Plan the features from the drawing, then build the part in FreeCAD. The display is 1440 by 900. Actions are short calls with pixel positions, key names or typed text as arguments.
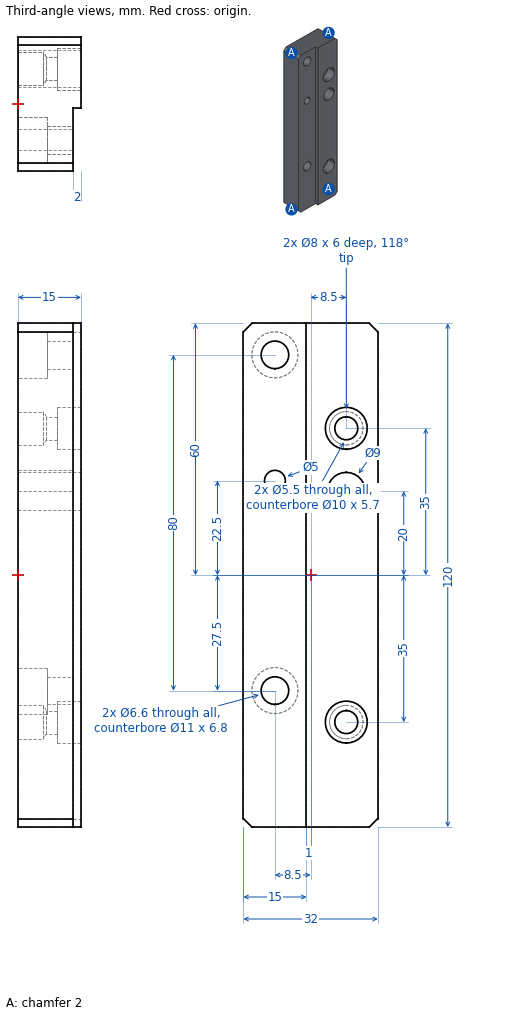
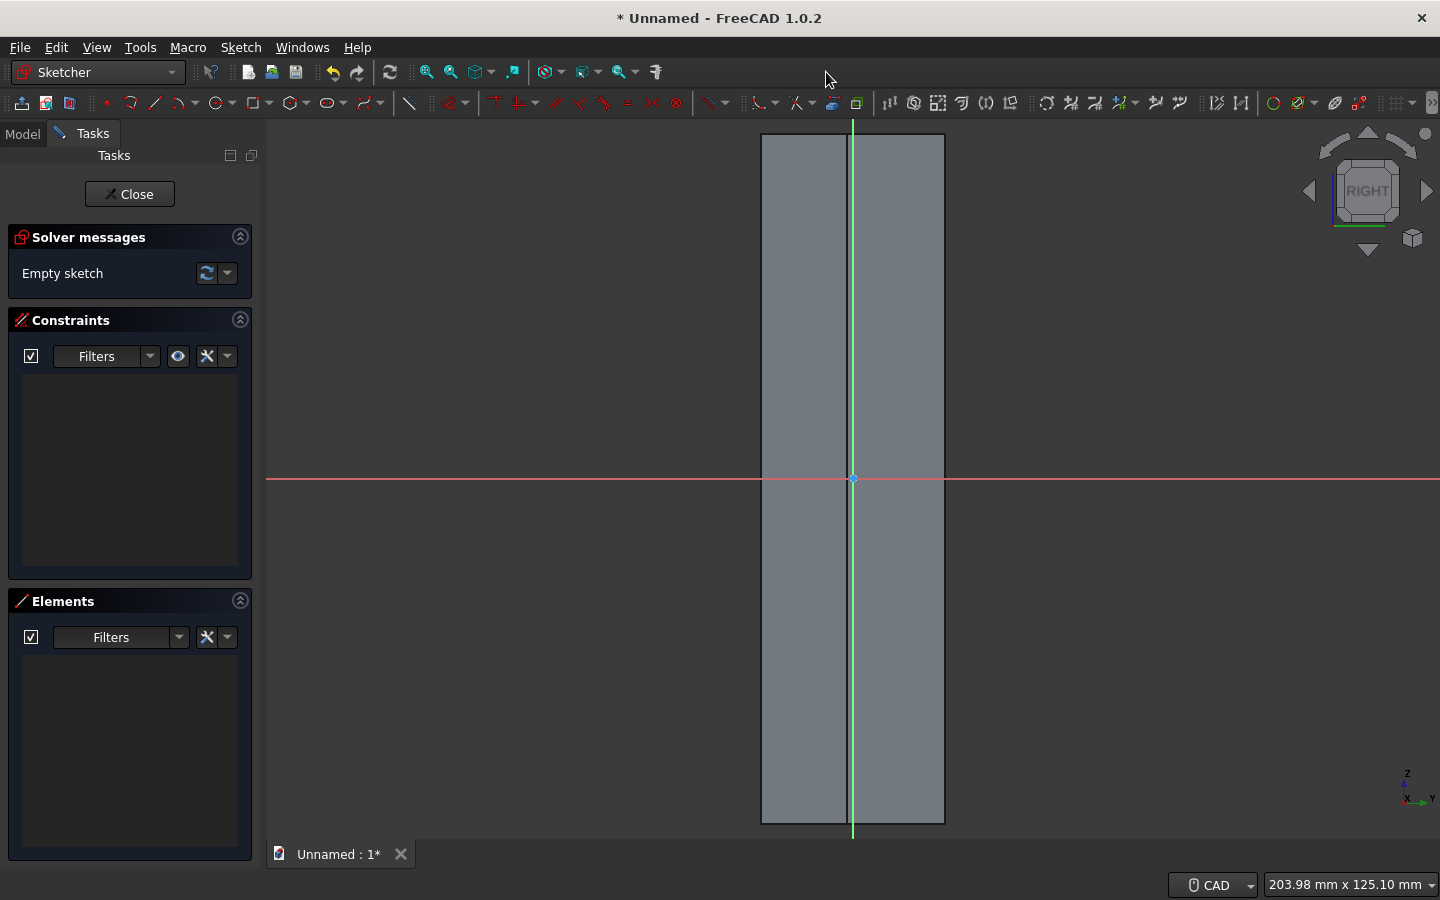
scroll(917, 350, up, 11)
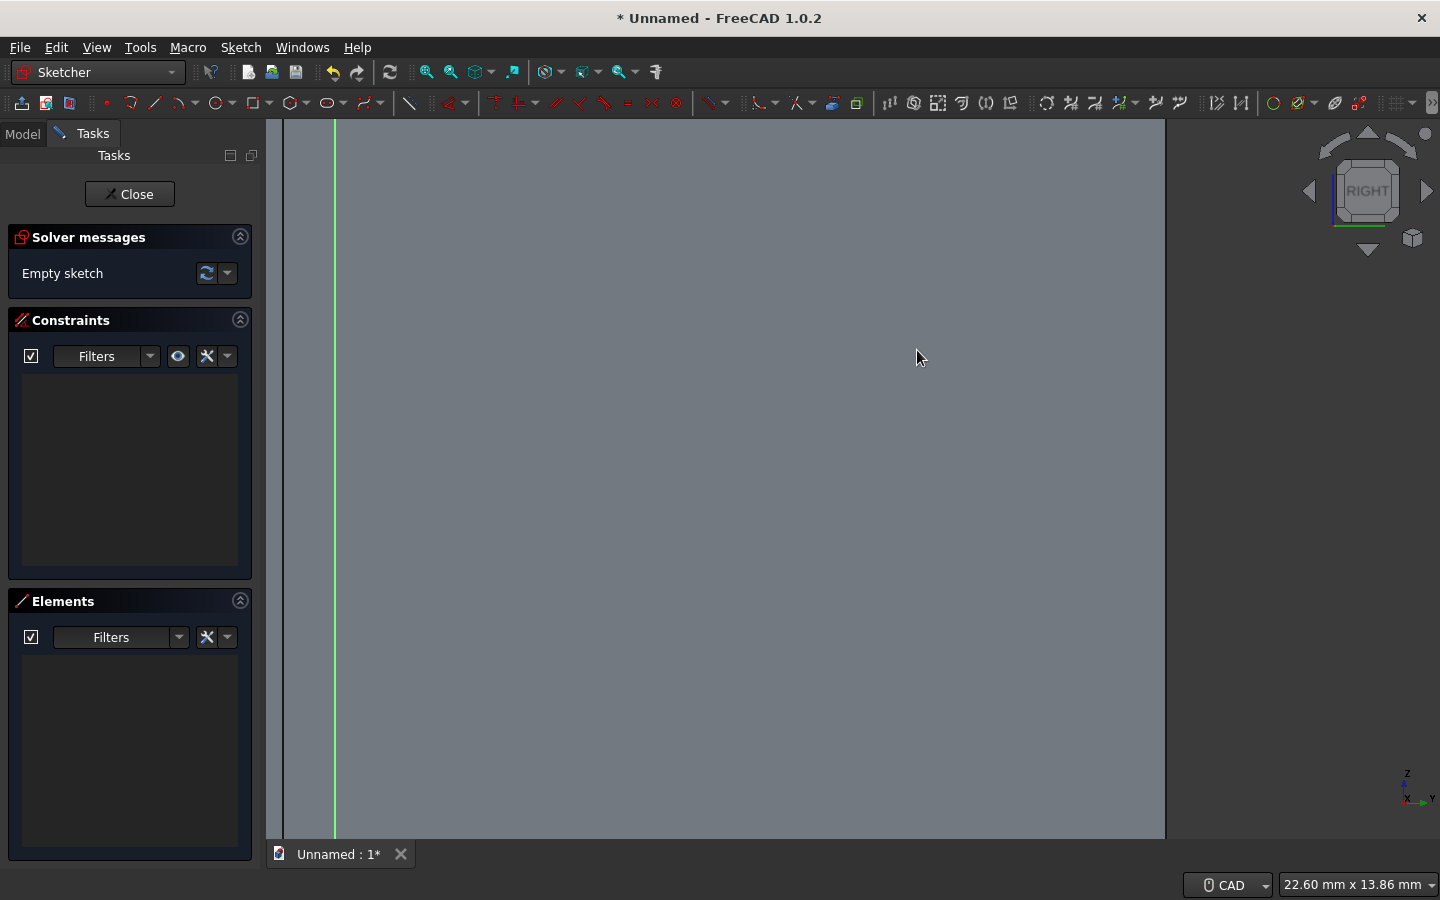
click(216, 104)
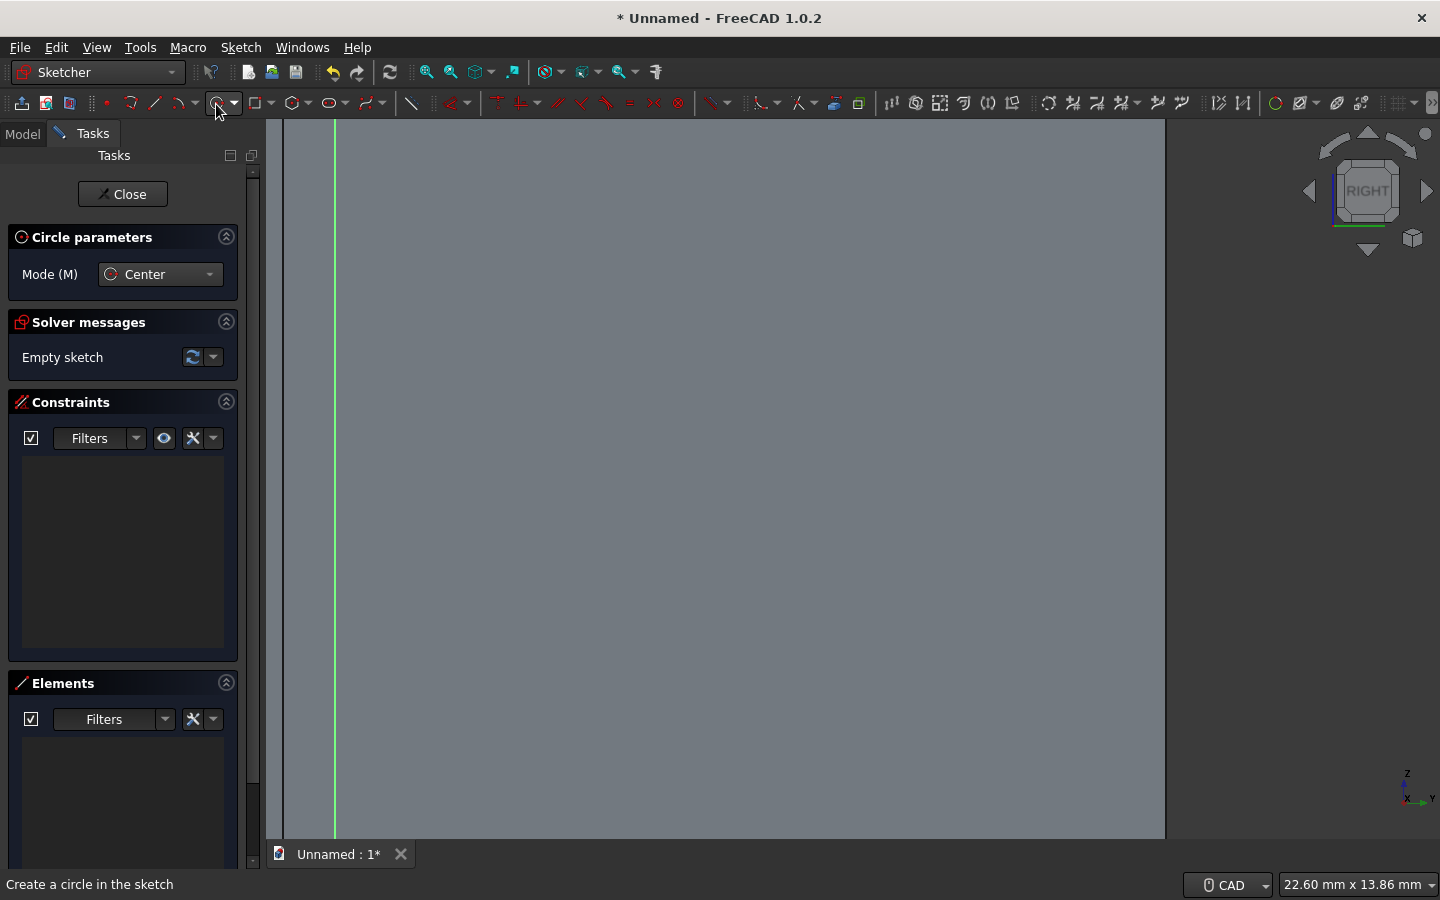
click(776, 473)
click(942, 307)
key(Escape)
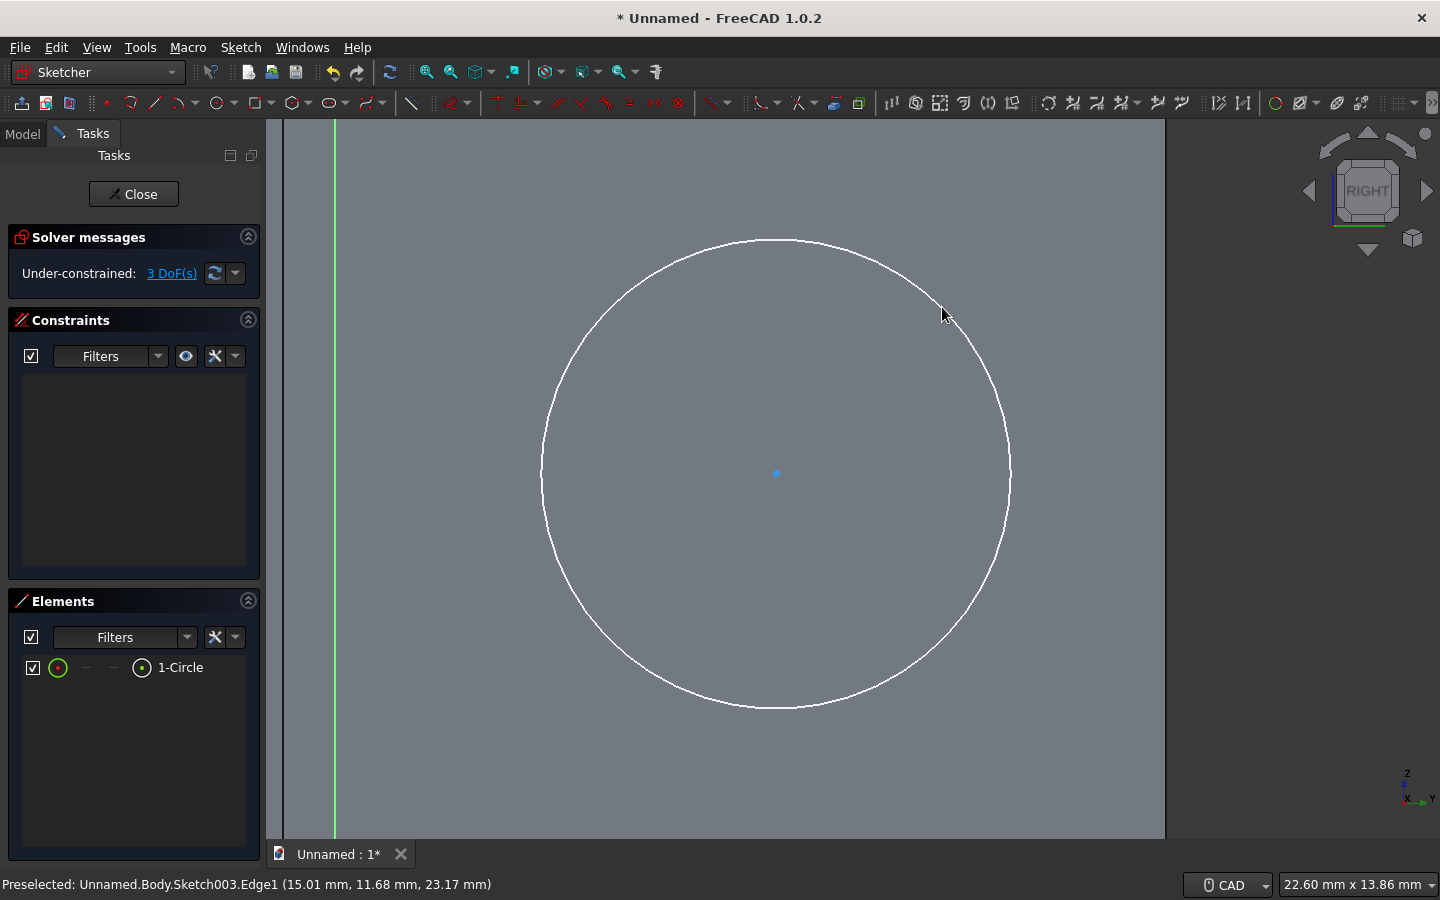
click(450, 104)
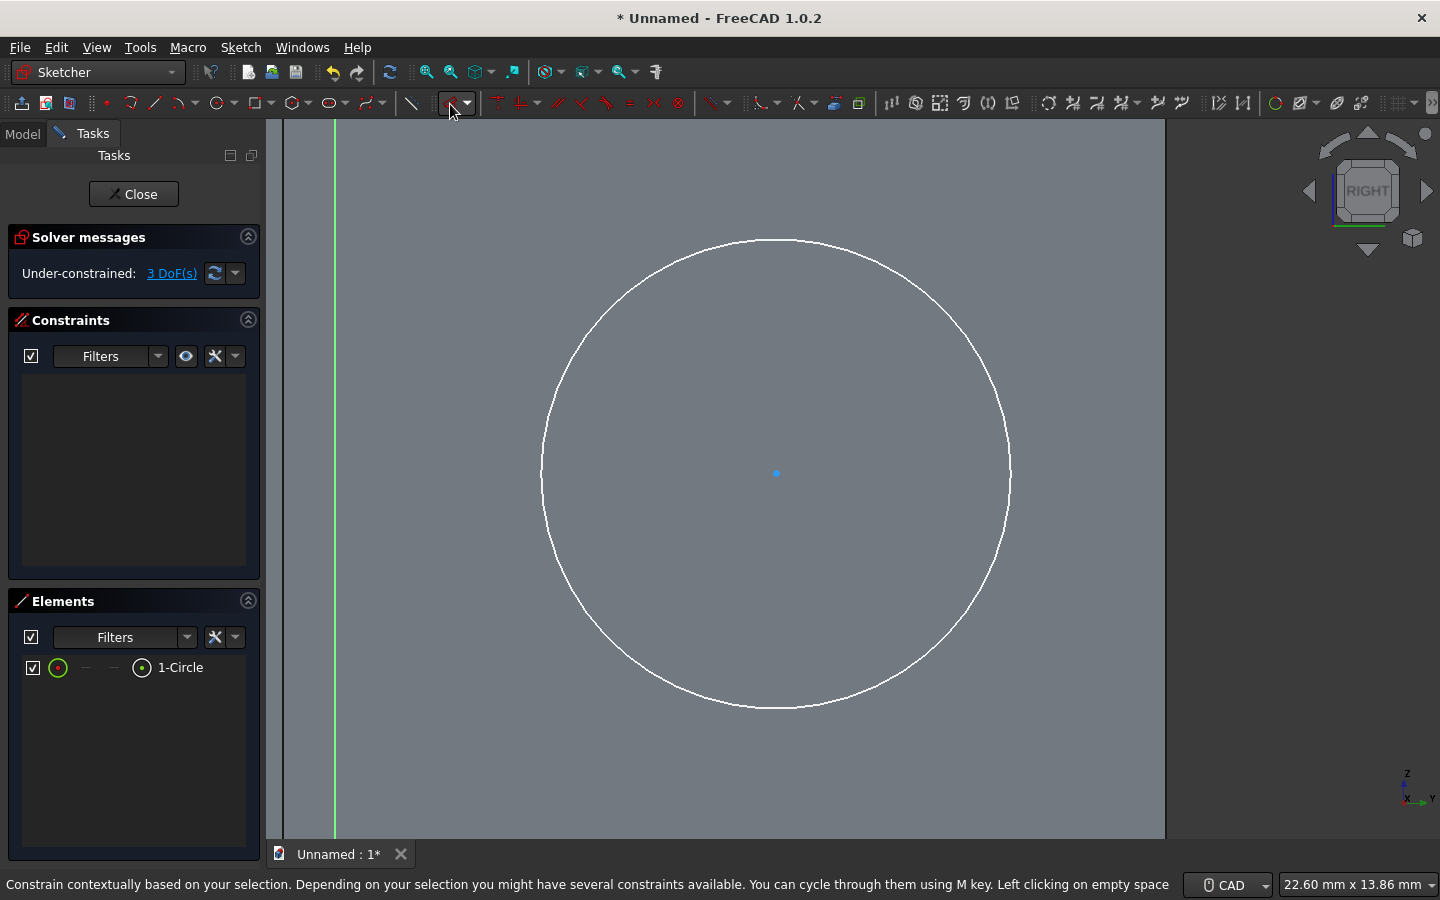
click(941, 307)
click(963, 284)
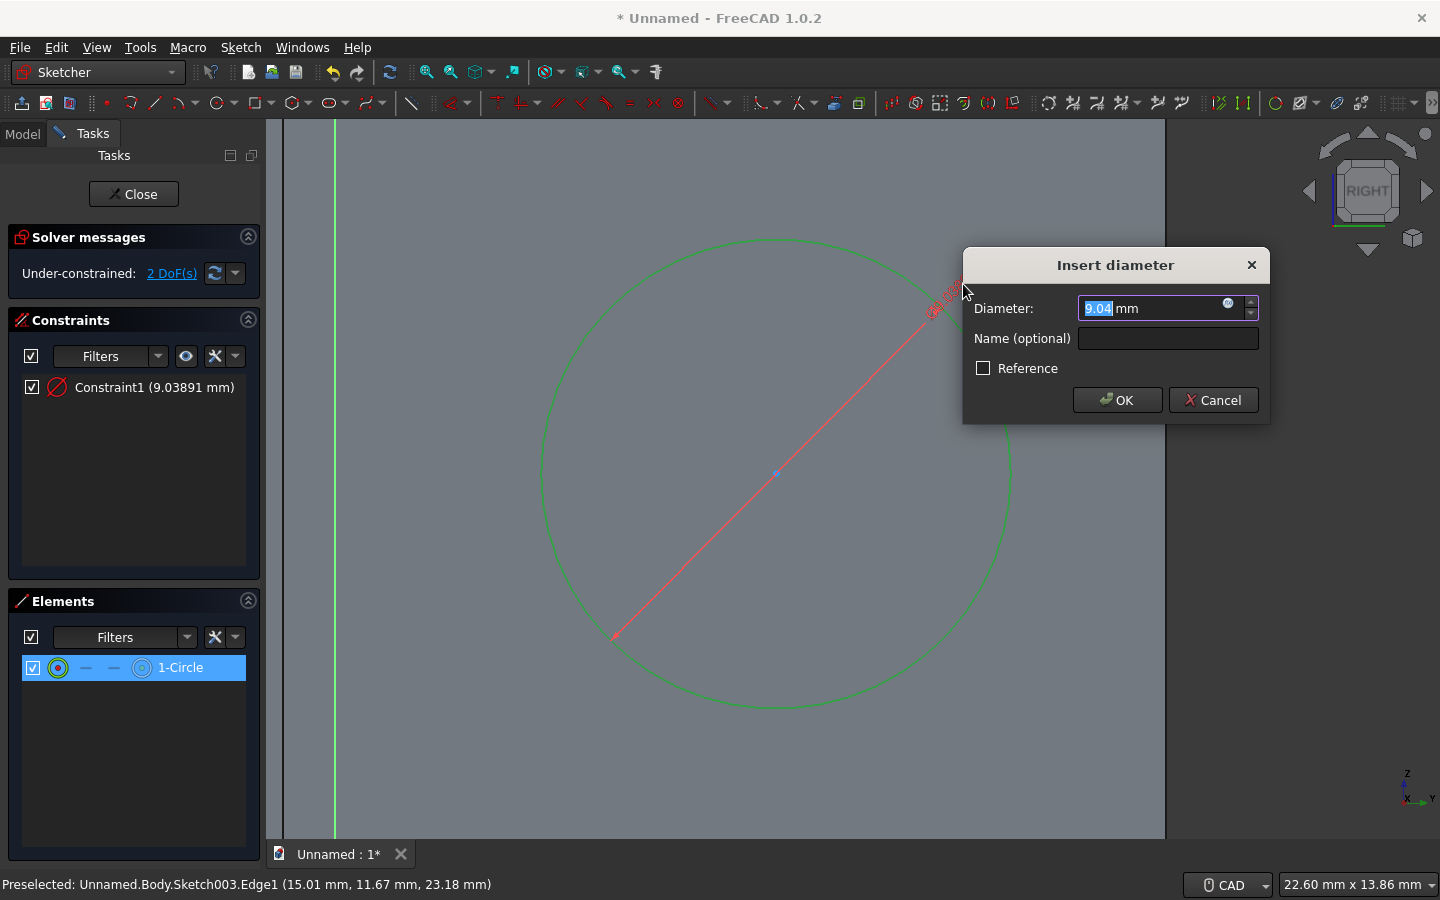
text(9)
key(Return)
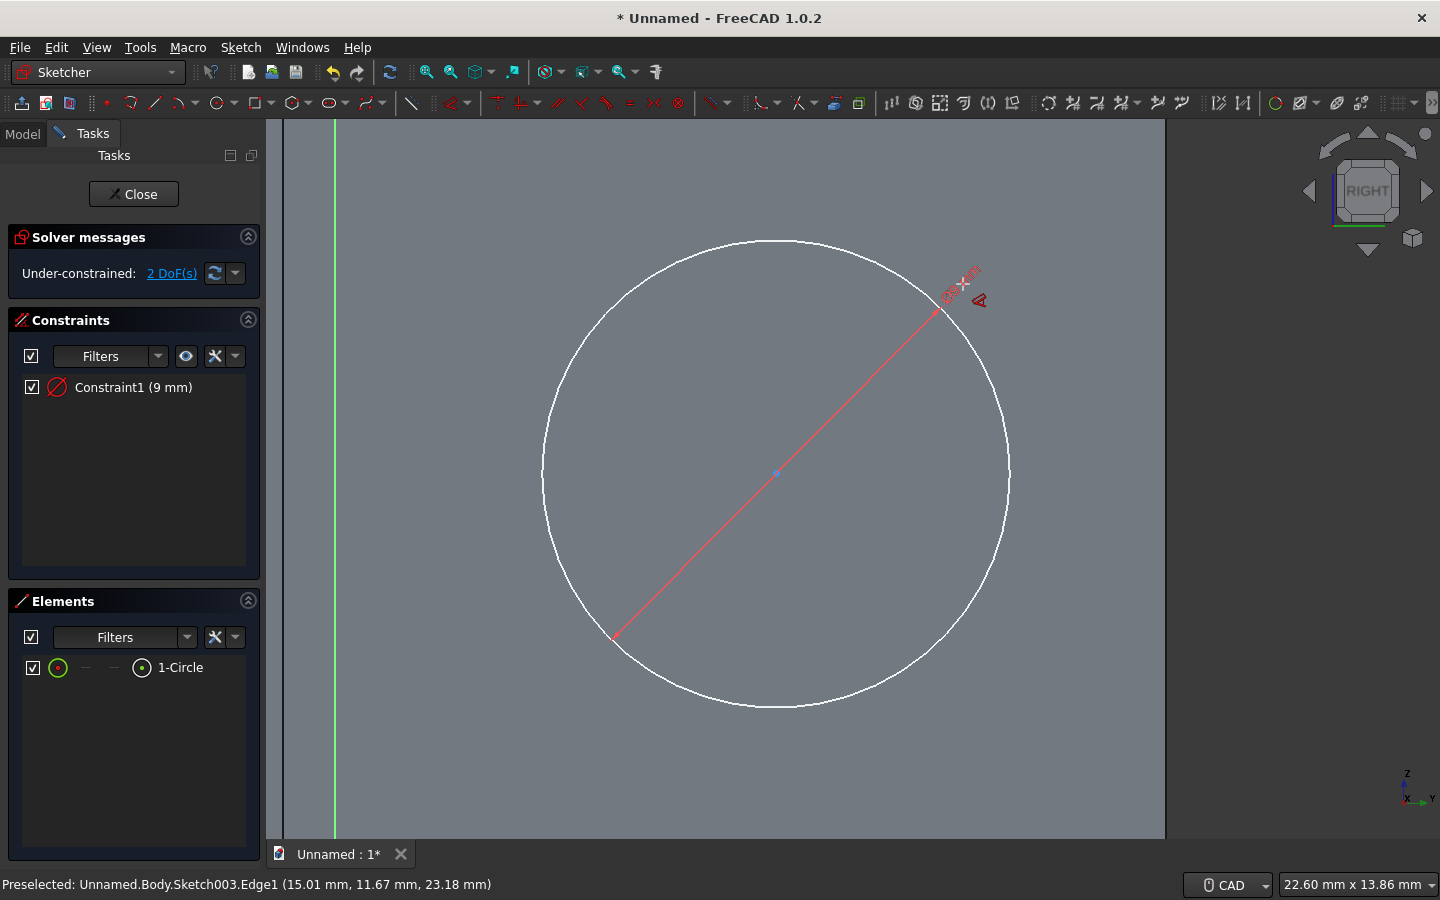
click(776, 474)
click(301, 643)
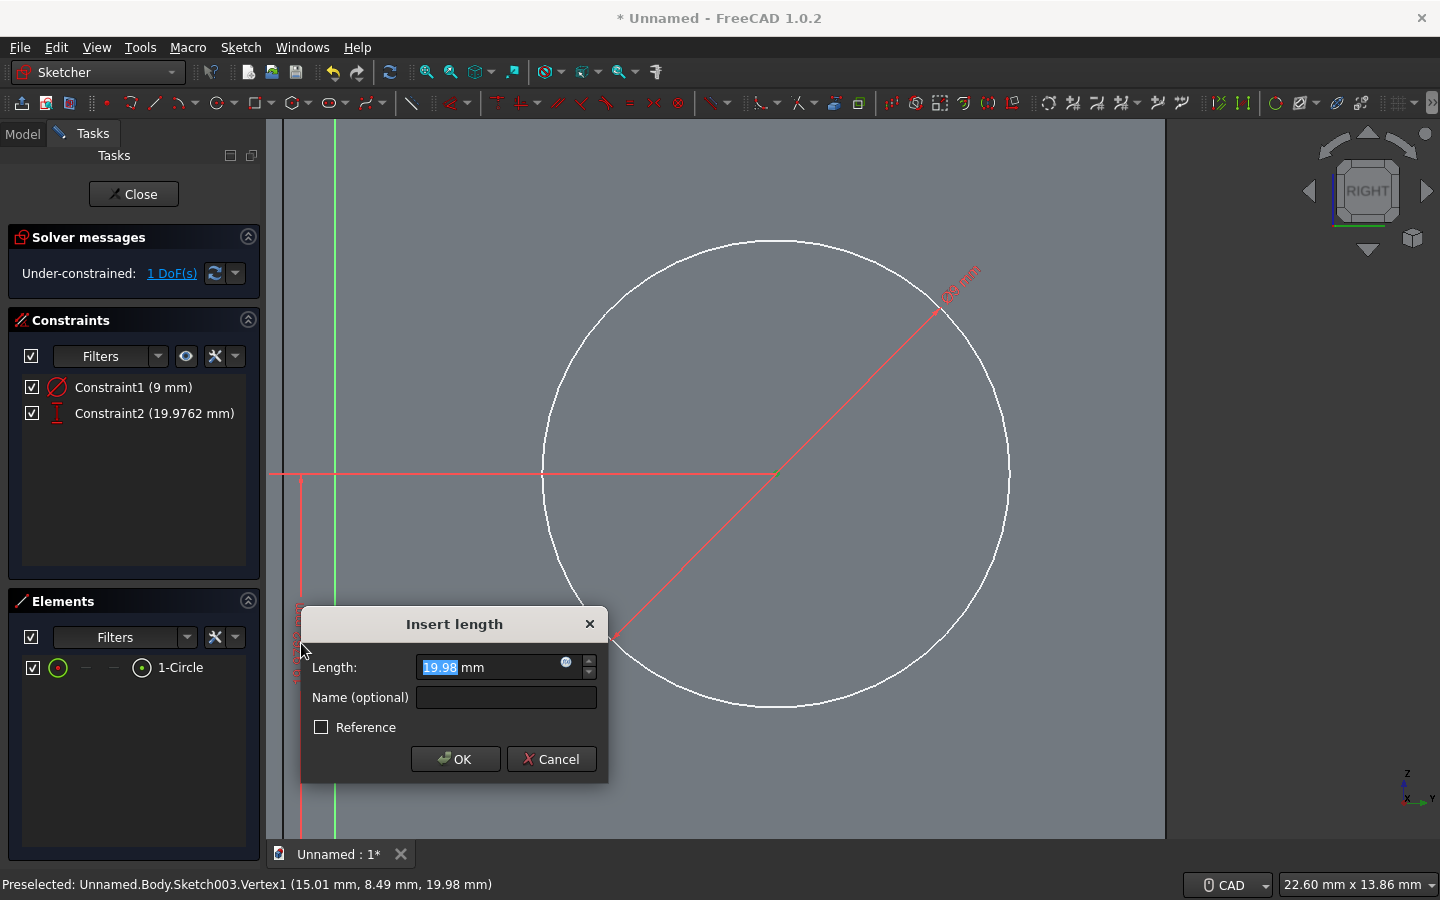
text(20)
key(Return)